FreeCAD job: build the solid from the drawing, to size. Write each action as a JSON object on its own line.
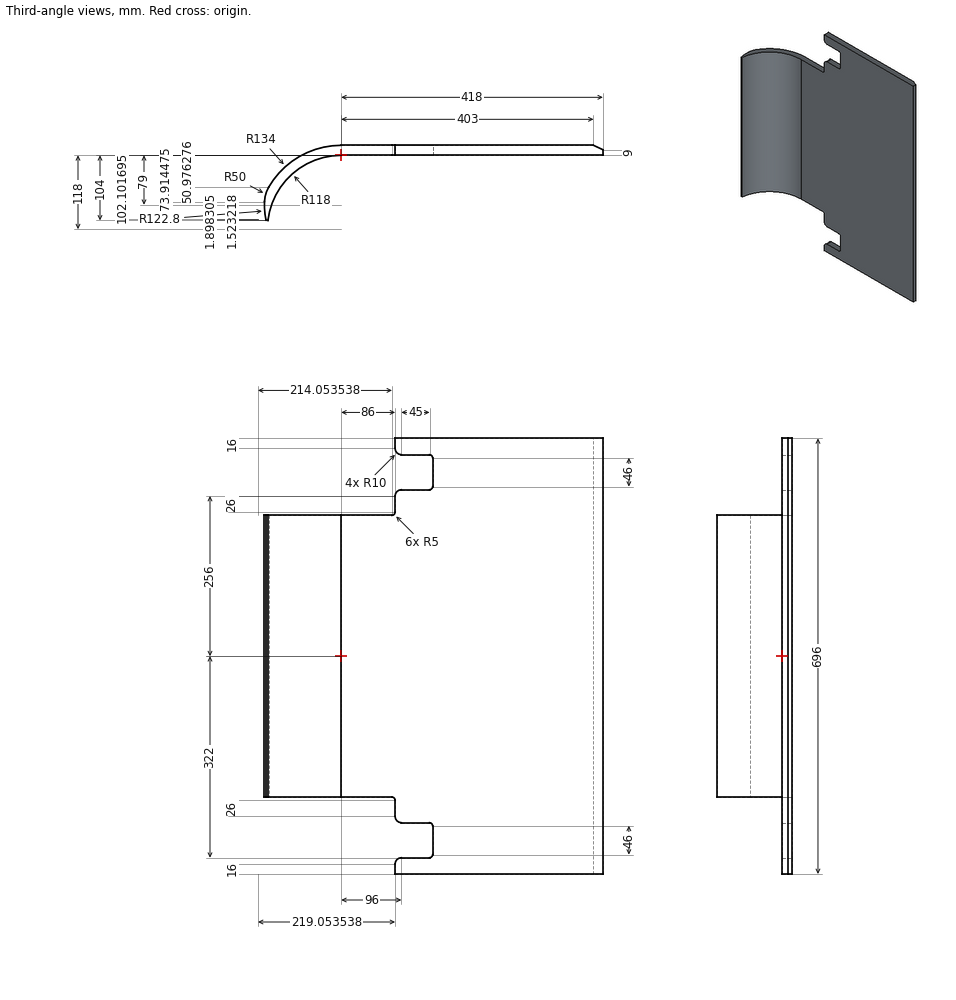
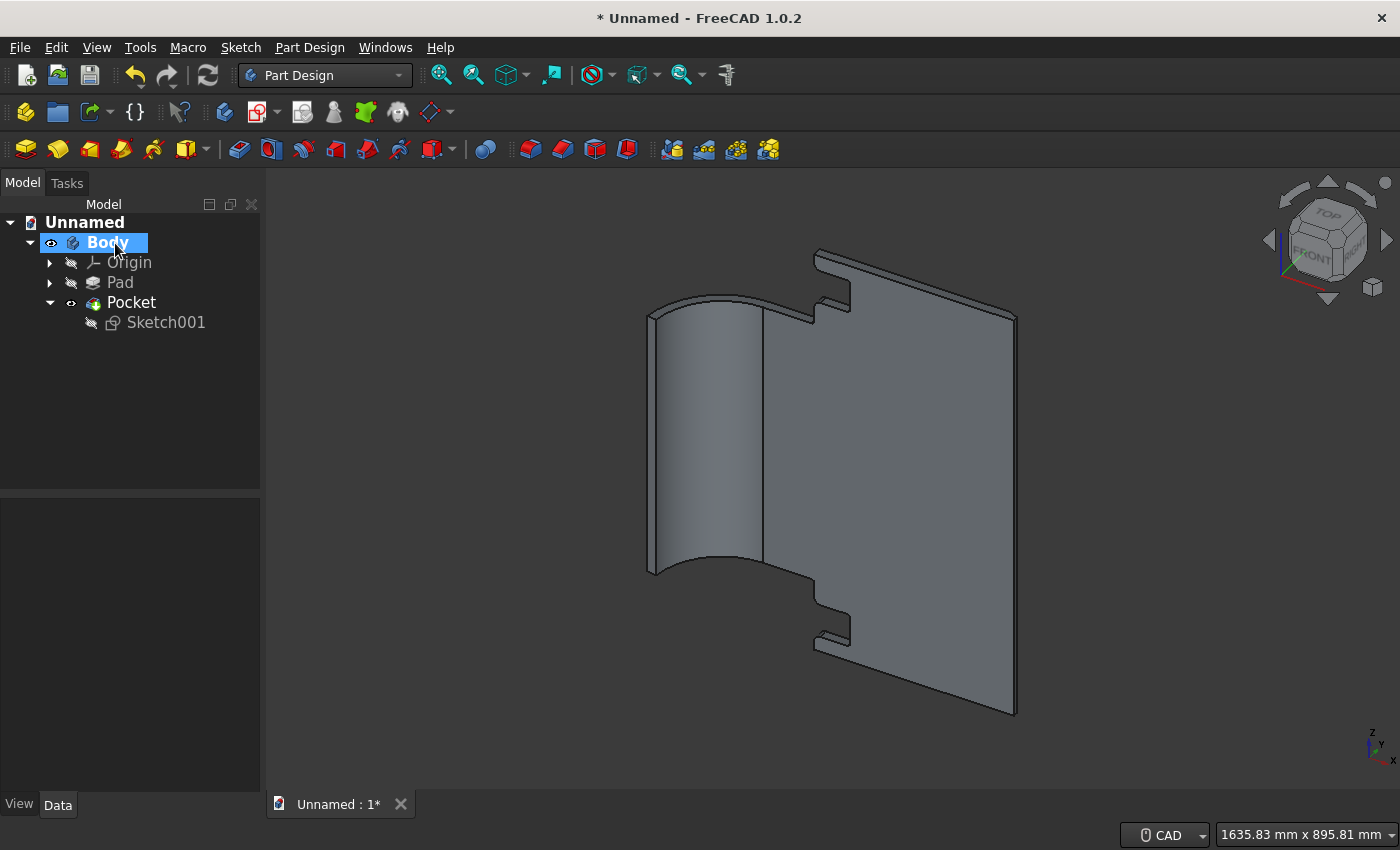
{"action": "scroll", "coordinate": [701, 298], "scroll_direction": "up", "scroll_amount": 4}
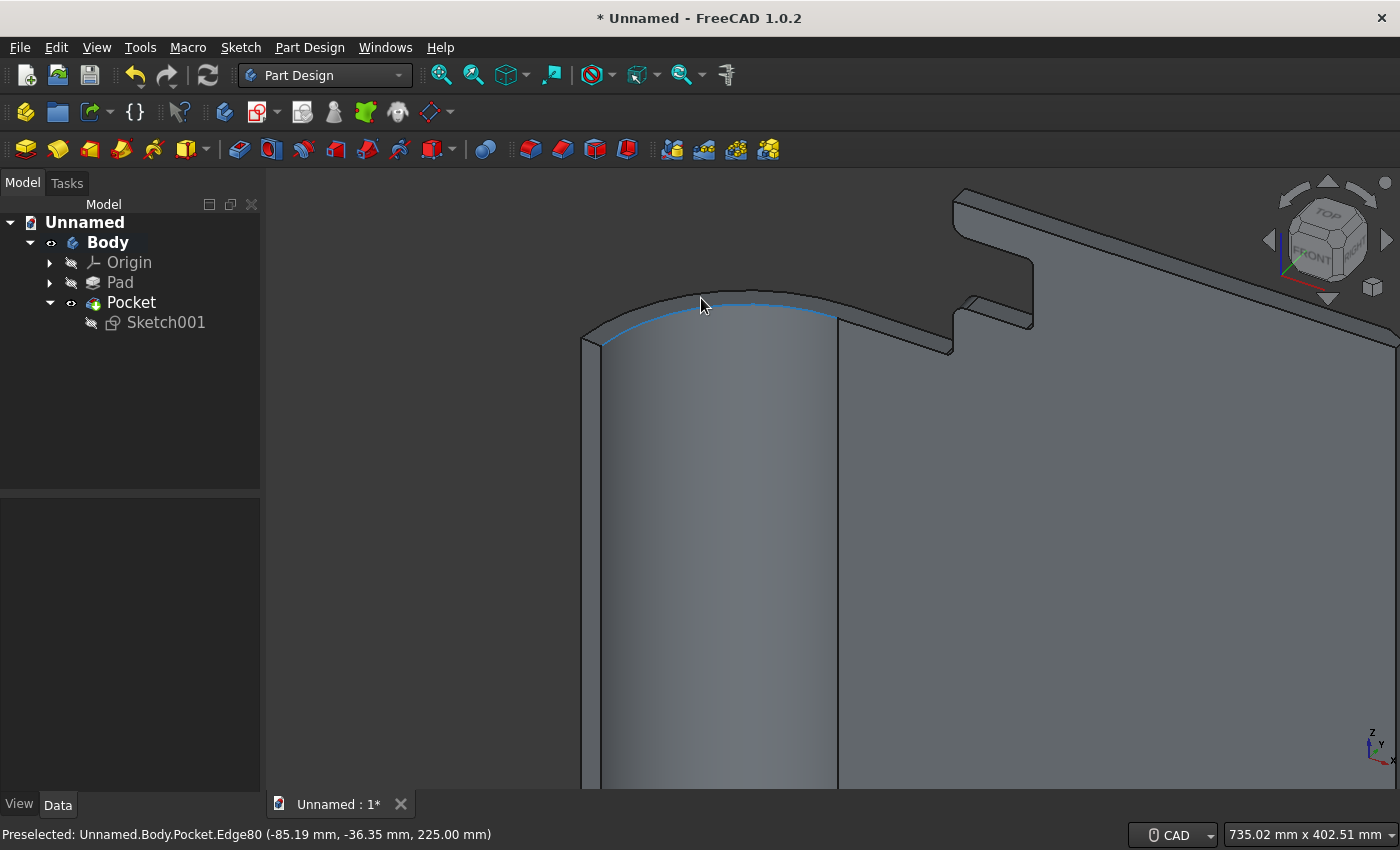
{"action": "left_click", "coordinate": [809, 300]}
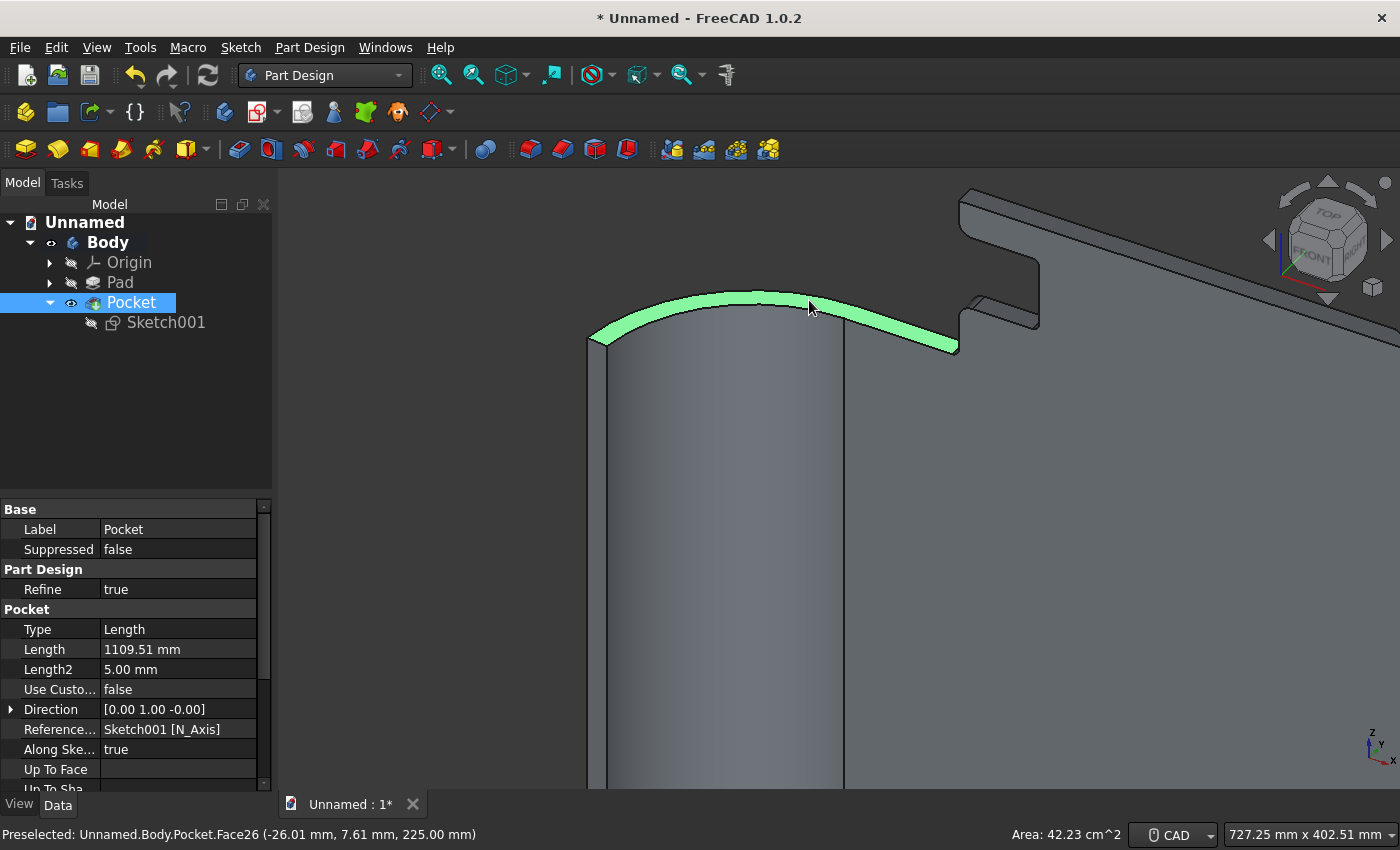
{"action": "left_click", "coordinate": [258, 112]}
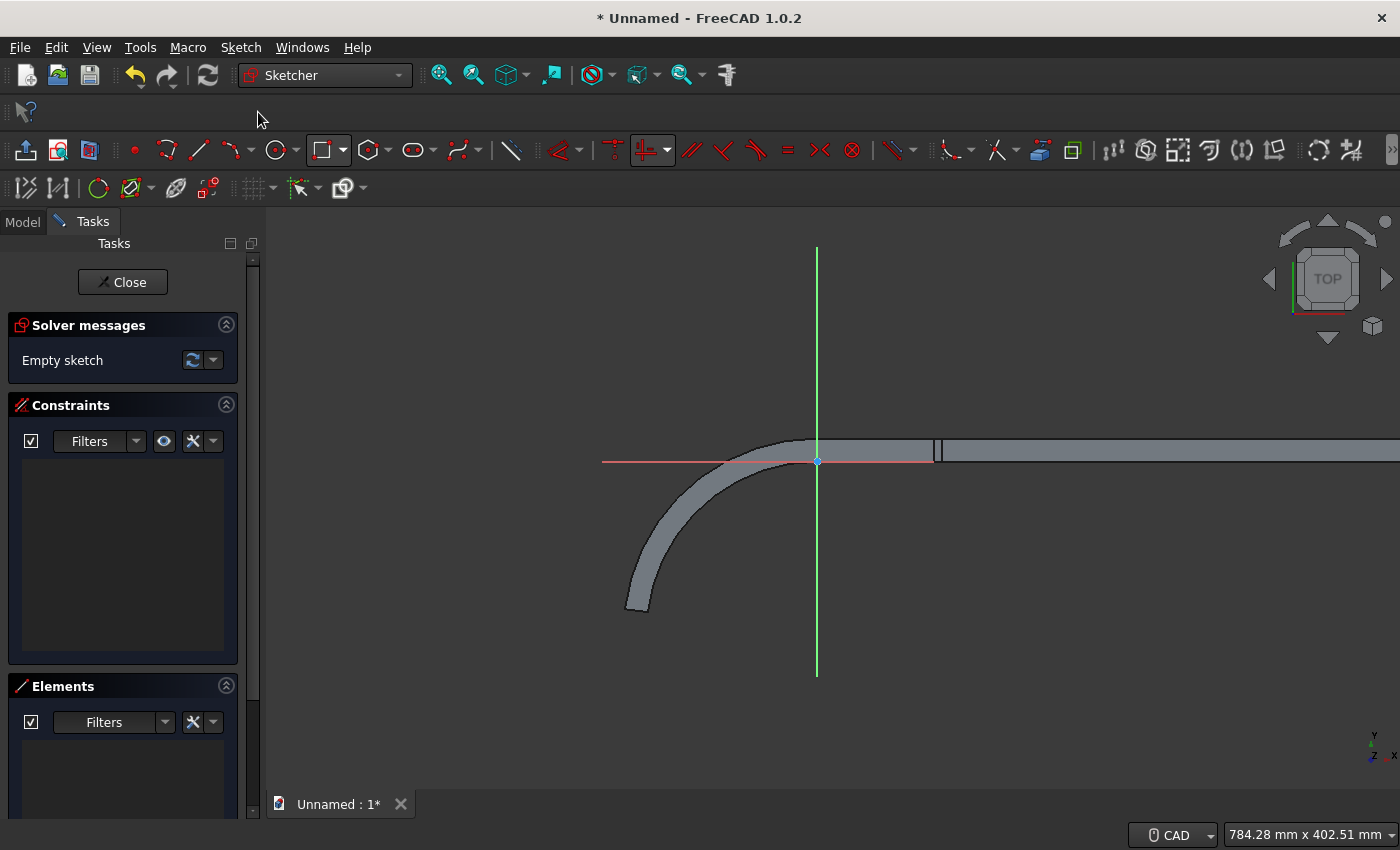
{"action": "scroll", "coordinate": [605, 593], "scroll_direction": "up", "scroll_amount": 8}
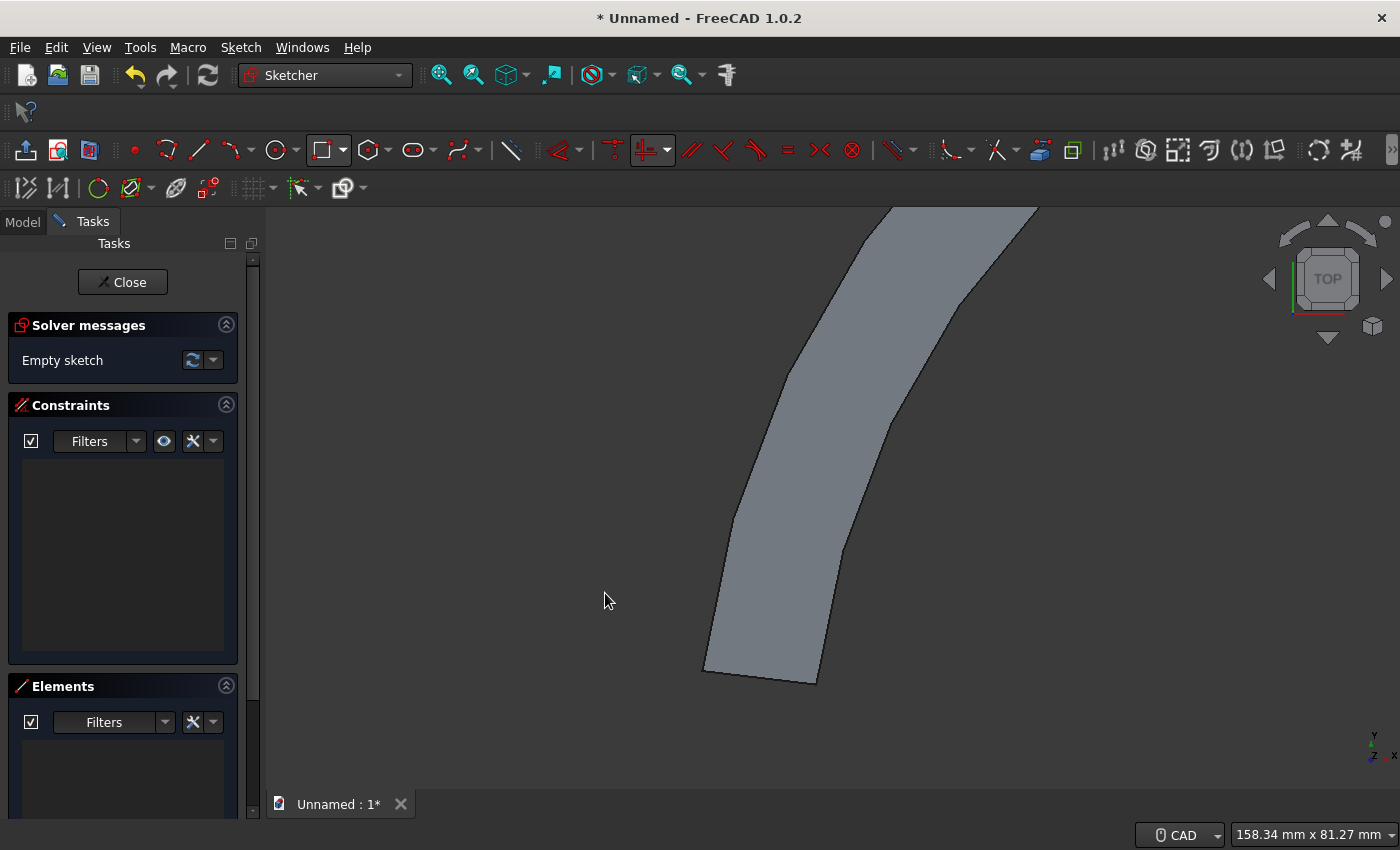
{"action": "left_click", "coordinate": [200, 150]}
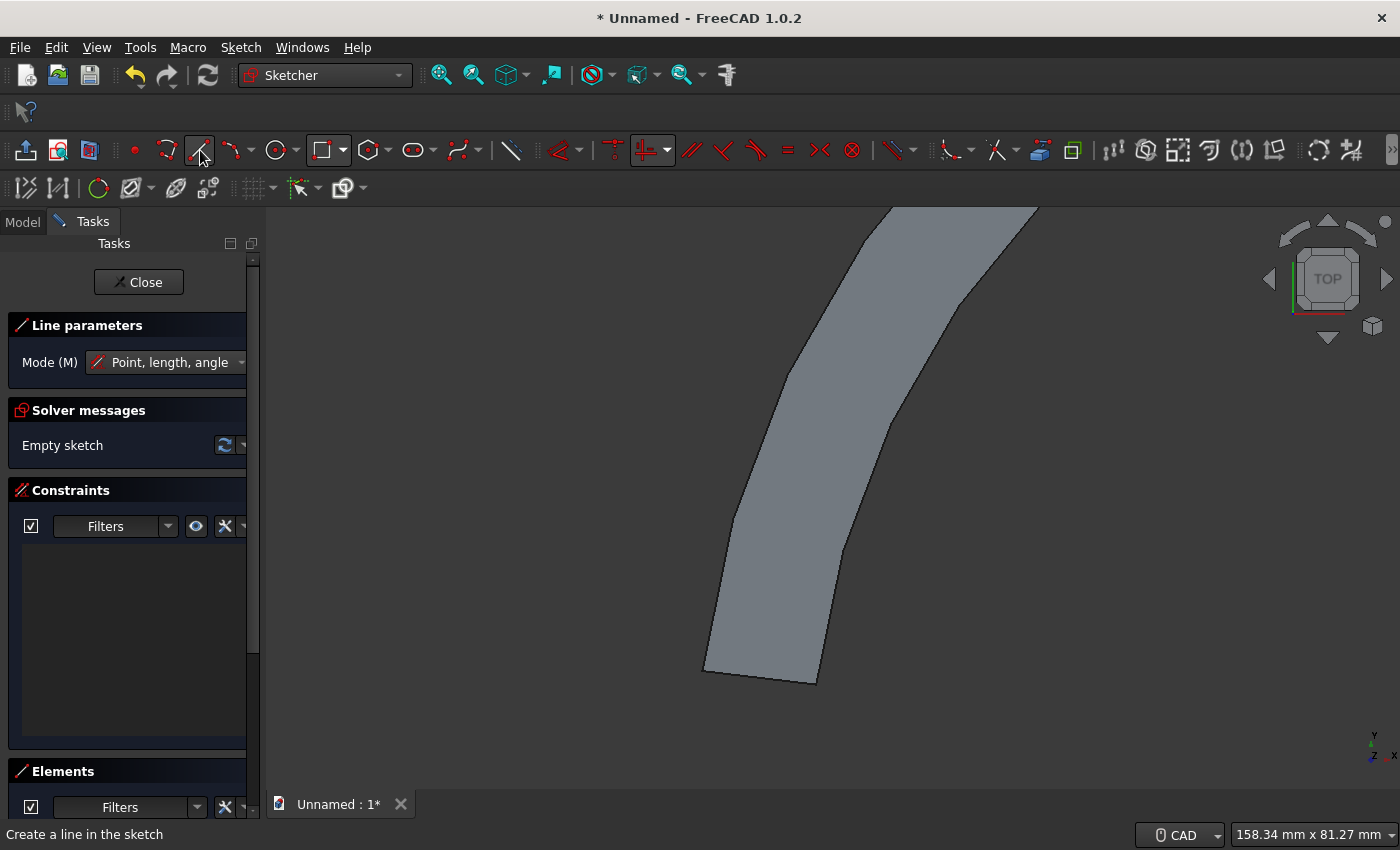
{"action": "left_click", "coordinate": [702, 671]}
{"action": "left_click", "coordinate": [794, 682]}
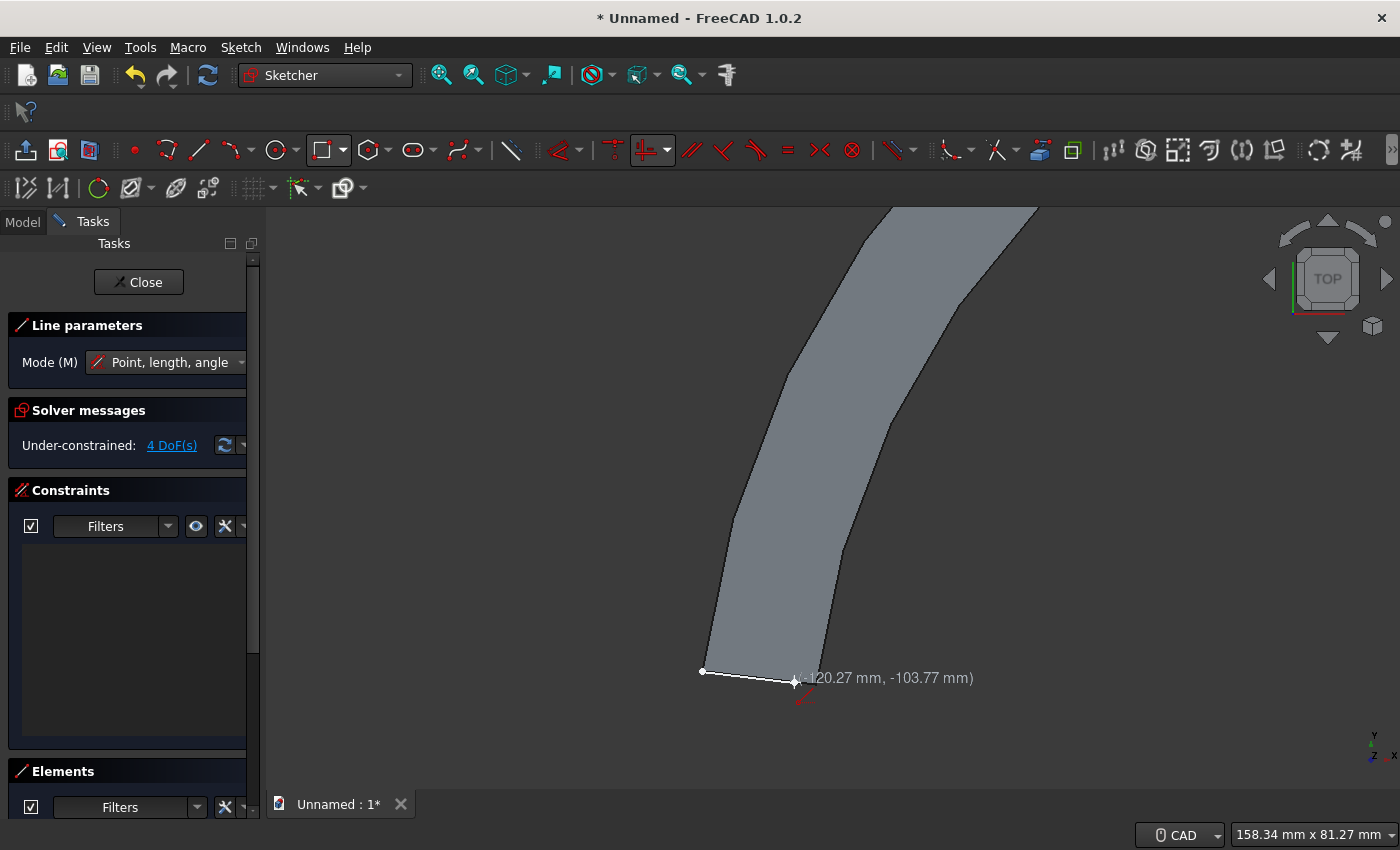
{"action": "left_click", "coordinate": [232, 150]}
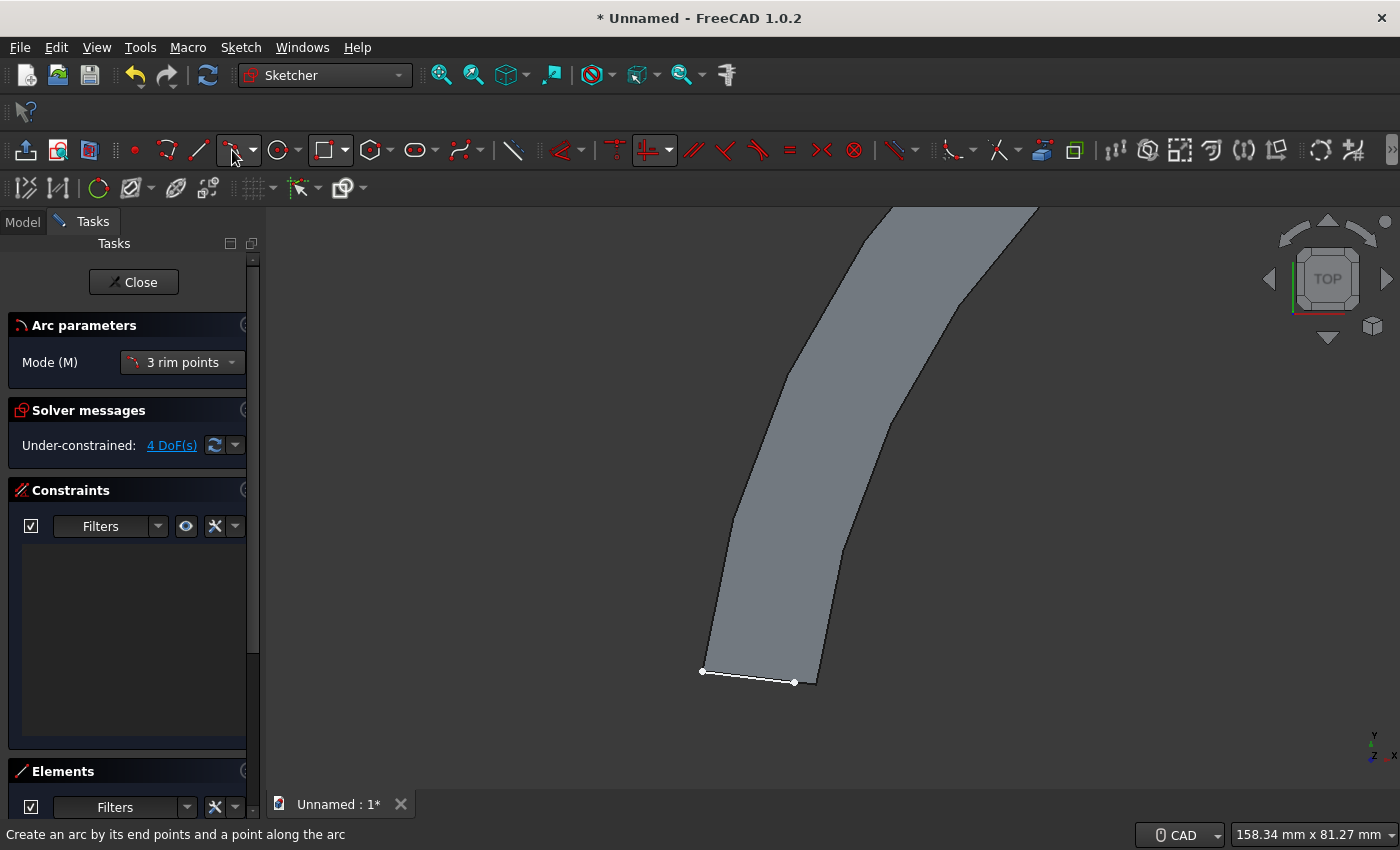
{"action": "left_click", "coordinate": [794, 683]}
{"action": "left_click", "coordinate": [777, 469]}